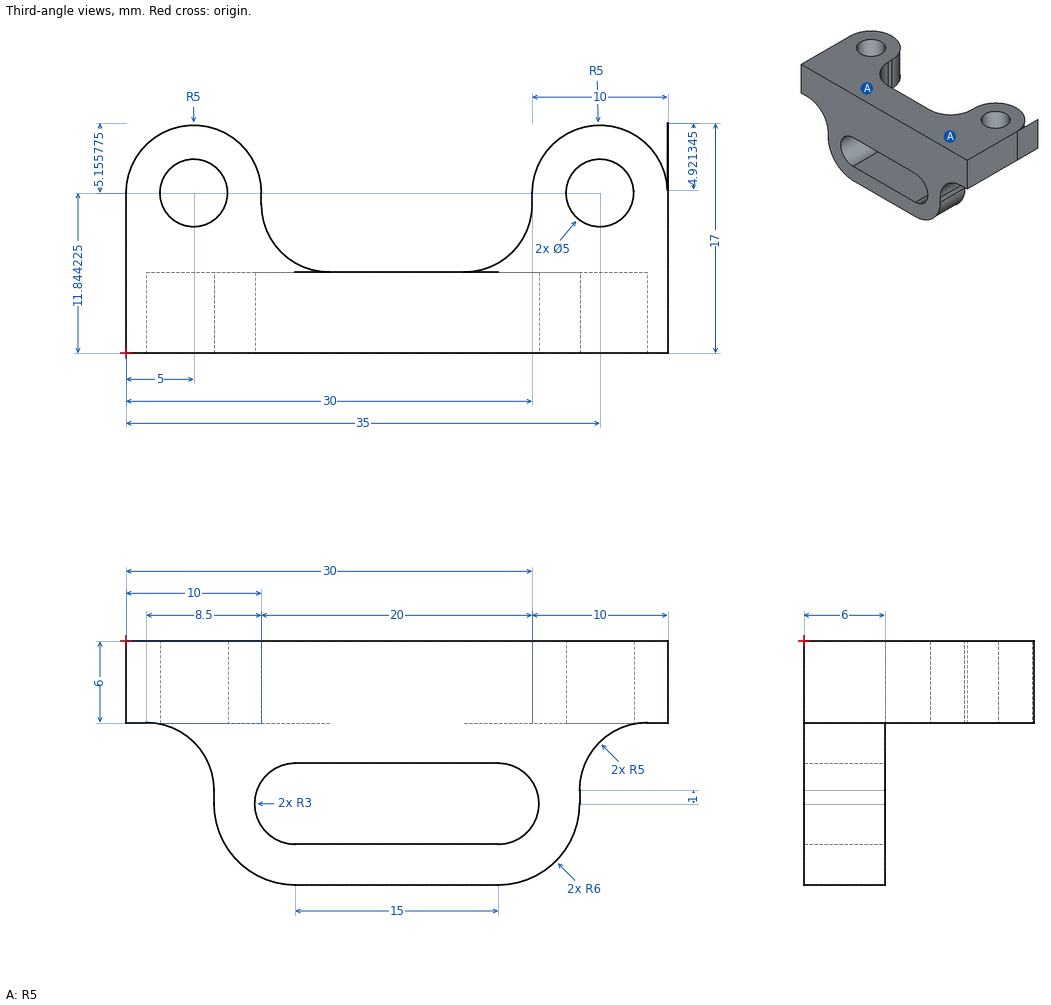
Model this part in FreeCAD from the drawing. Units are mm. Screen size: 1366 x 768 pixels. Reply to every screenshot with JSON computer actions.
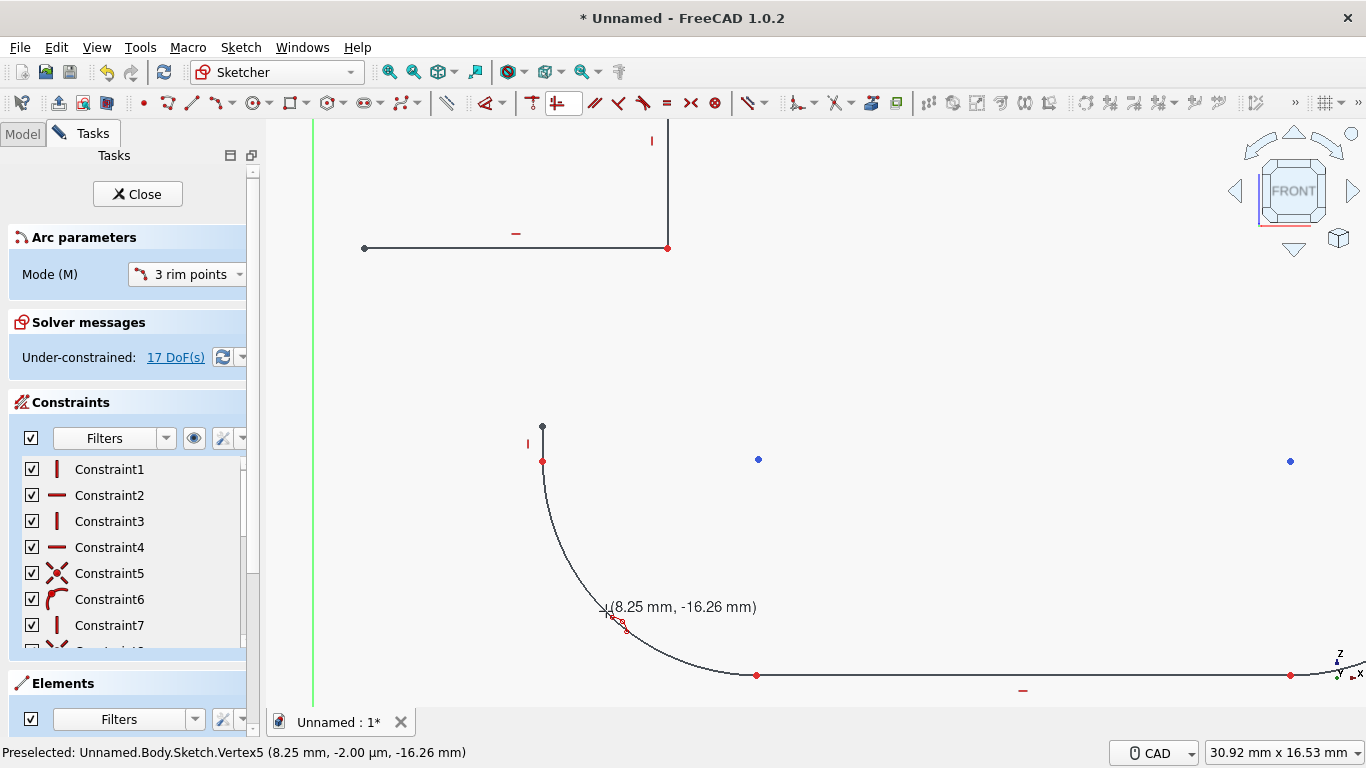
{"action": "left_click", "coordinate": [543, 426]}
{"action": "left_click", "coordinate": [365, 248]}
{"action": "left_click", "coordinate": [492, 299]}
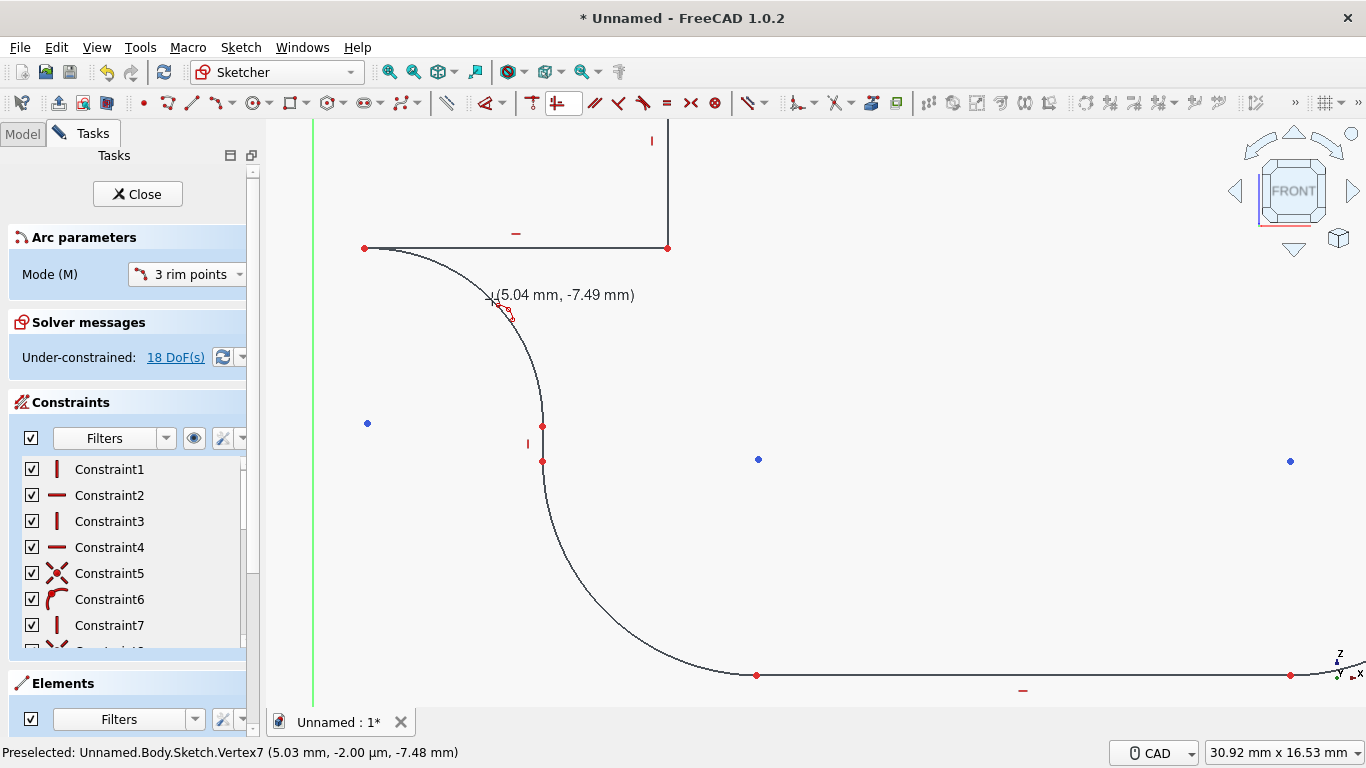
{"action": "scroll", "coordinate": [544, 461], "scroll_direction": "down", "scroll_amount": 4}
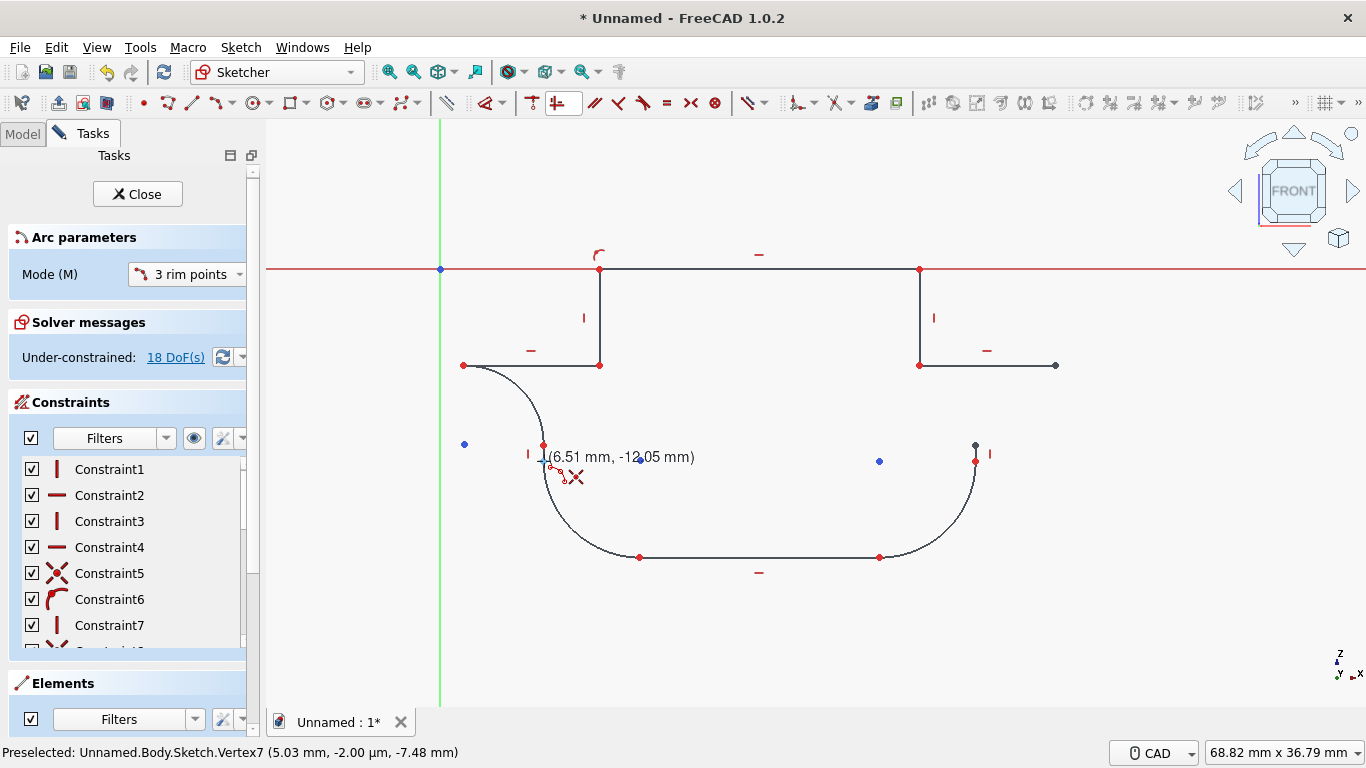
{"action": "left_click", "coordinate": [1056, 366]}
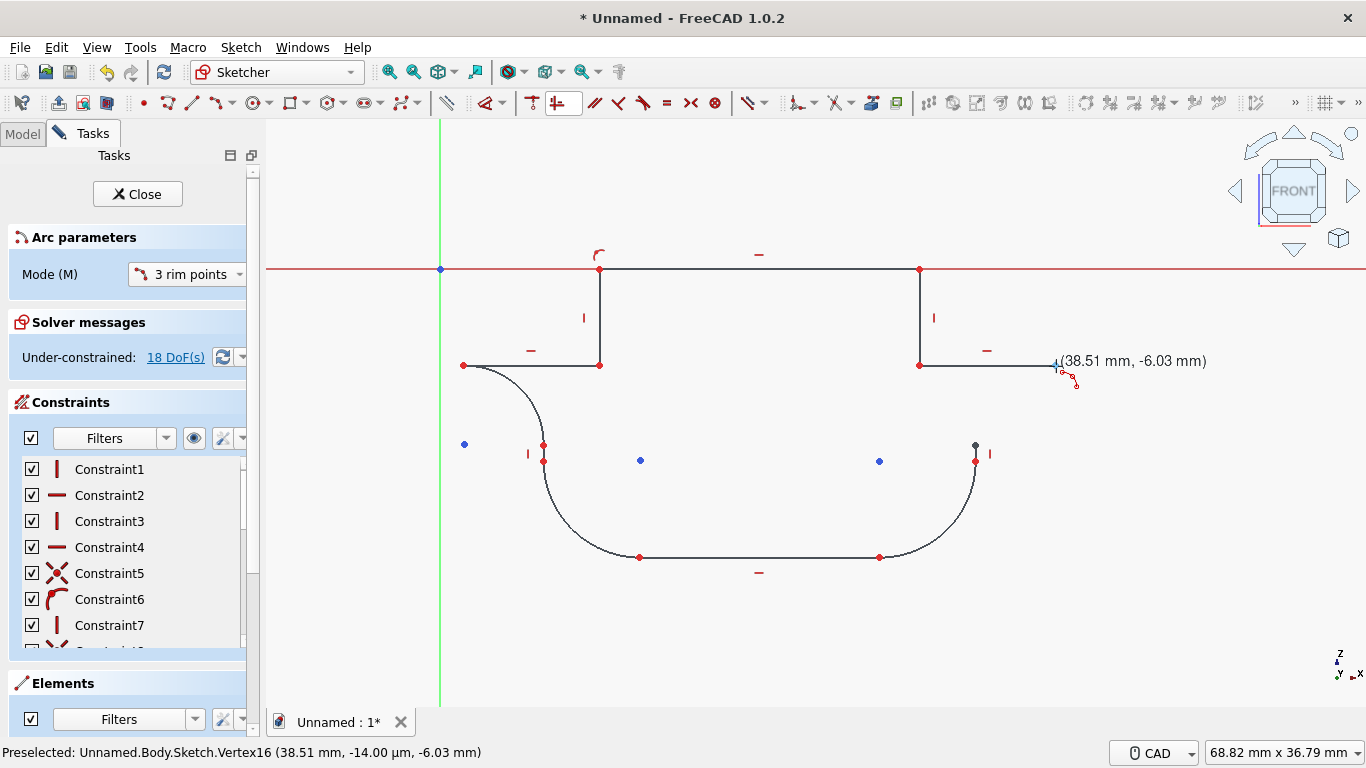
{"action": "scroll", "coordinate": [976, 445], "scroll_direction": "up", "scroll_amount": 4}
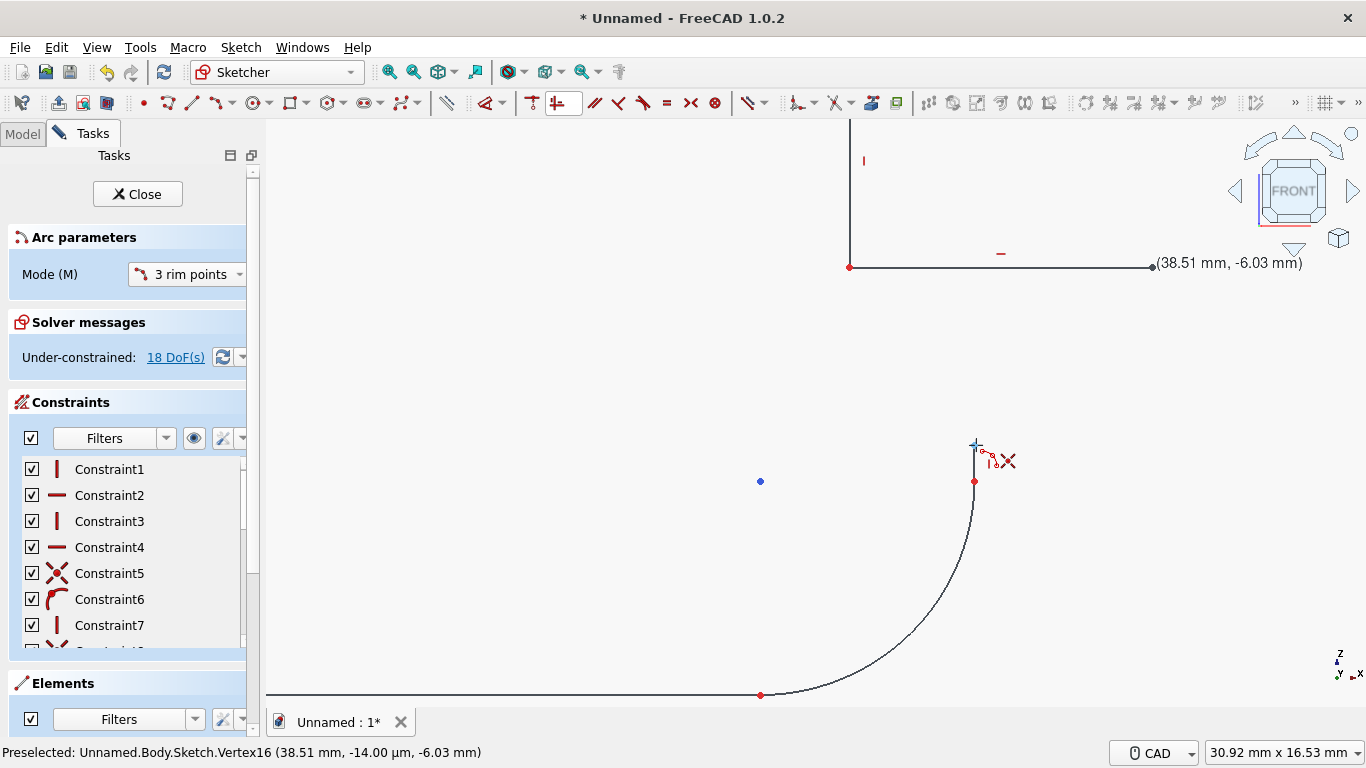
{"action": "left_click", "coordinate": [974, 446]}
{"action": "left_click", "coordinate": [1026, 319]}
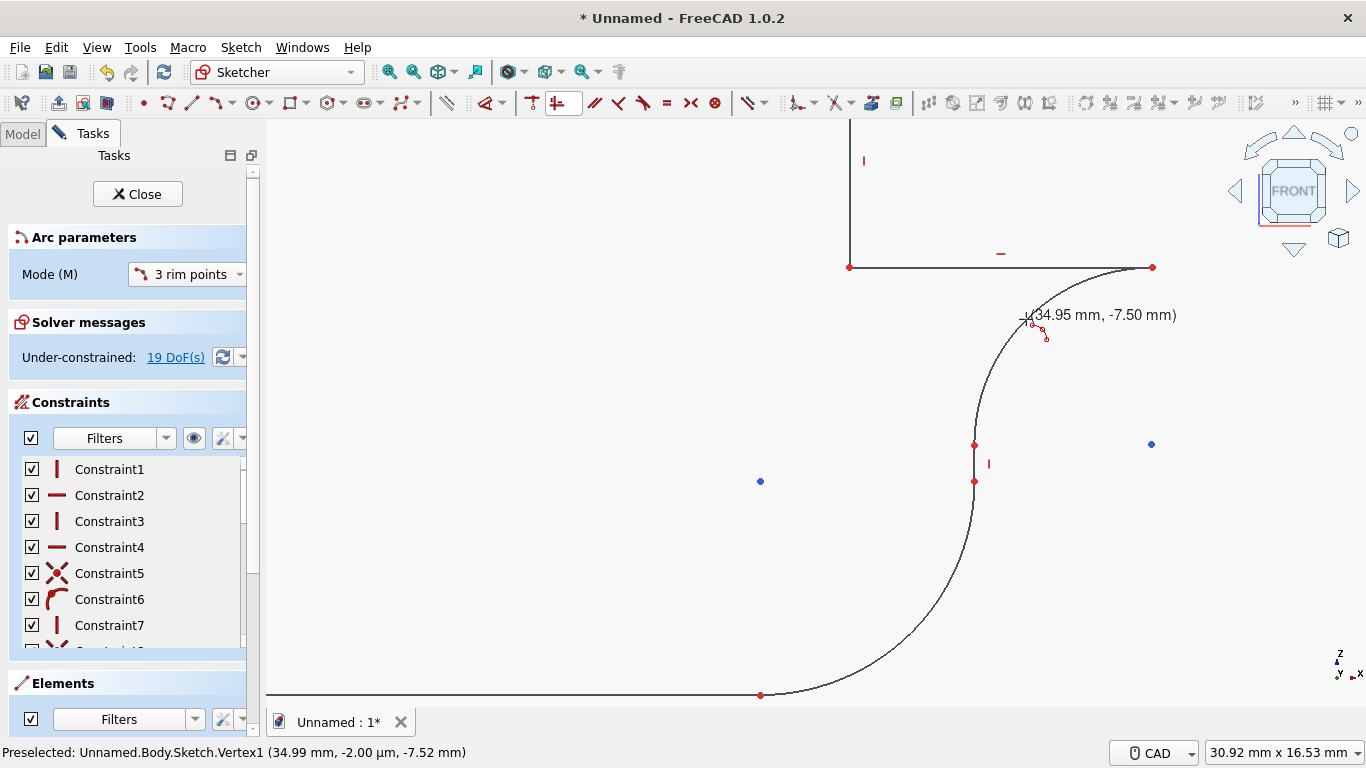
{"action": "left_click", "coordinate": [364, 104]}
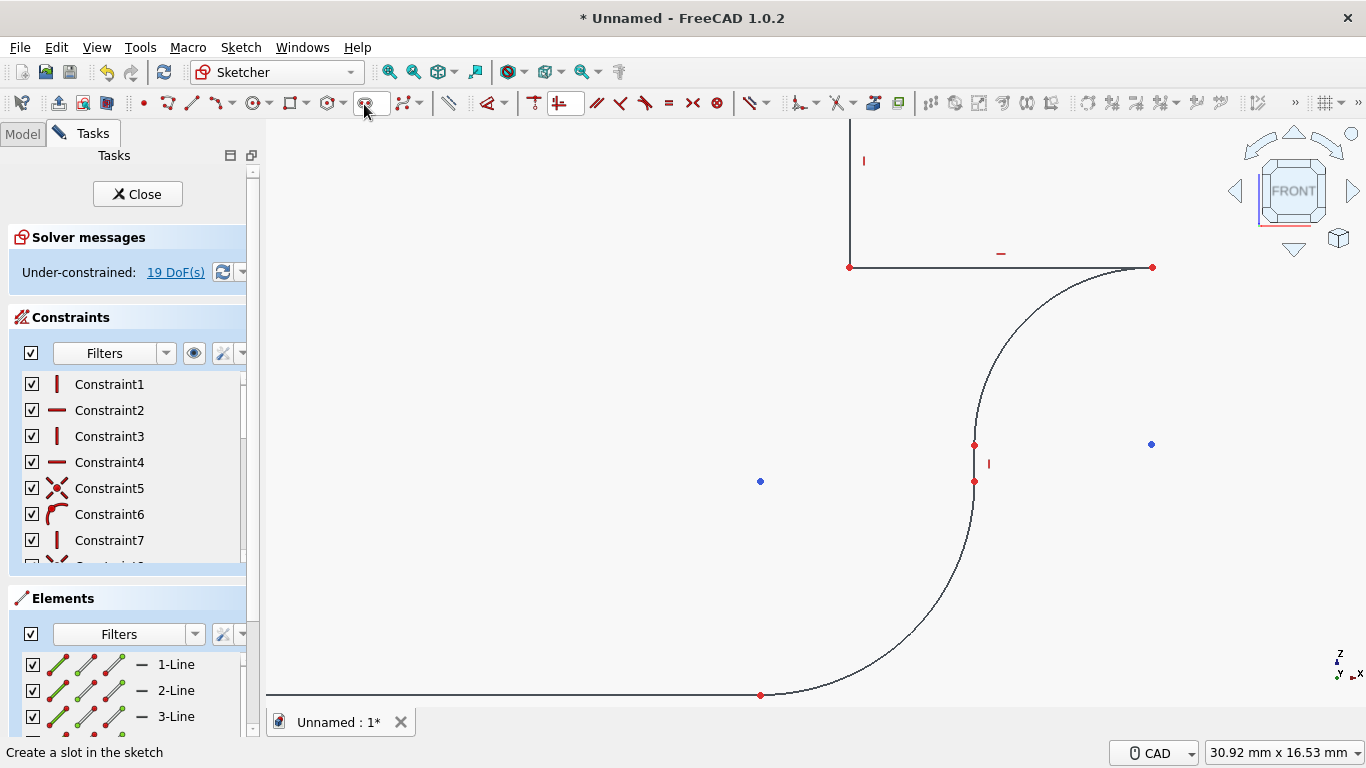
{"action": "scroll", "coordinate": [976, 445], "scroll_direction": "down", "scroll_amount": 4}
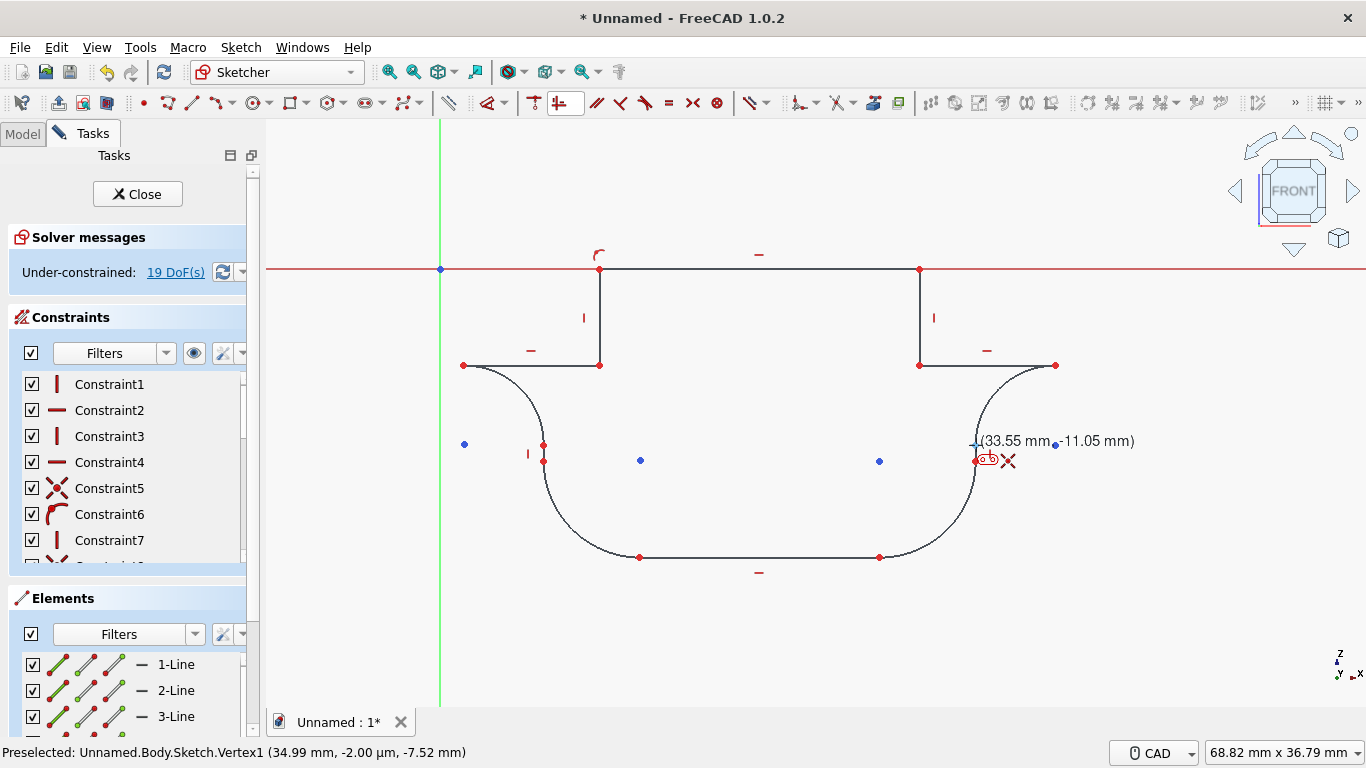
{"action": "left_click", "coordinate": [640, 461]}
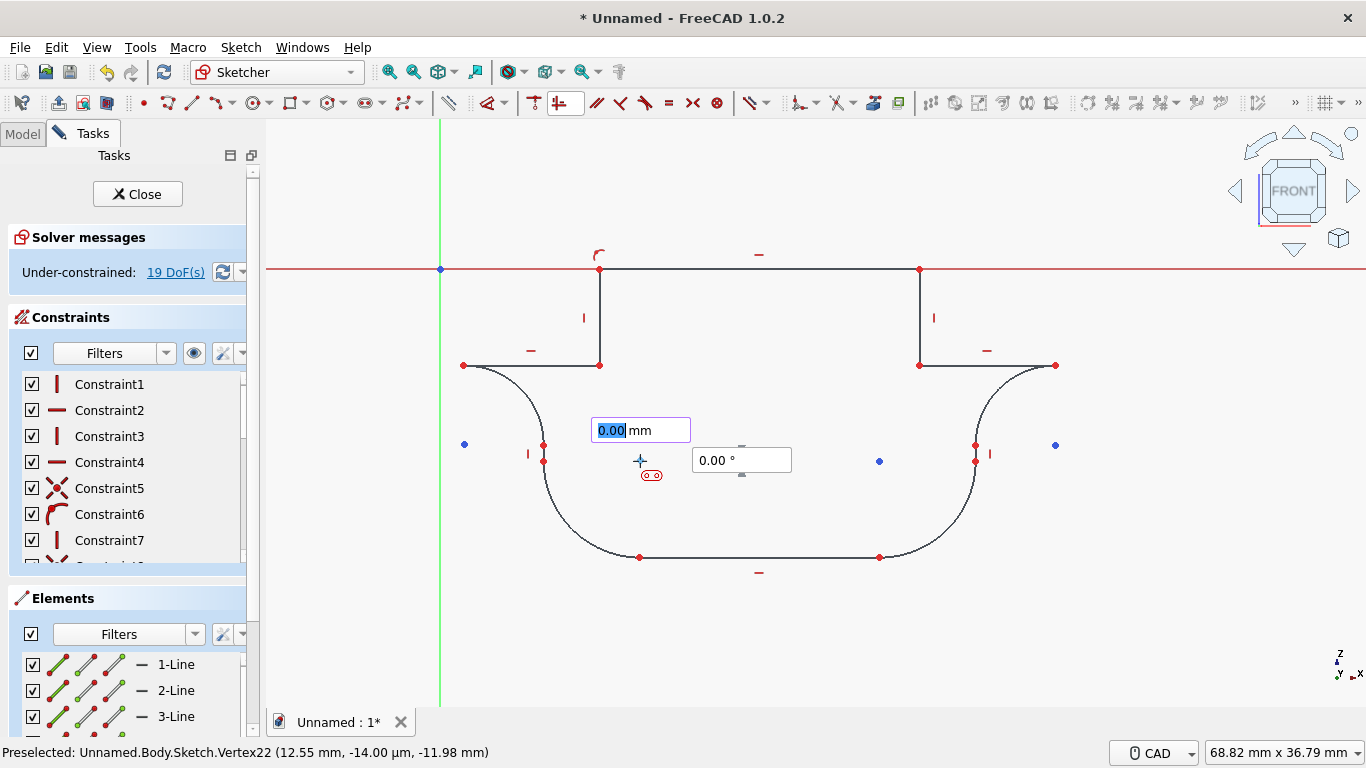
{"action": "left_click", "coordinate": [880, 461]}